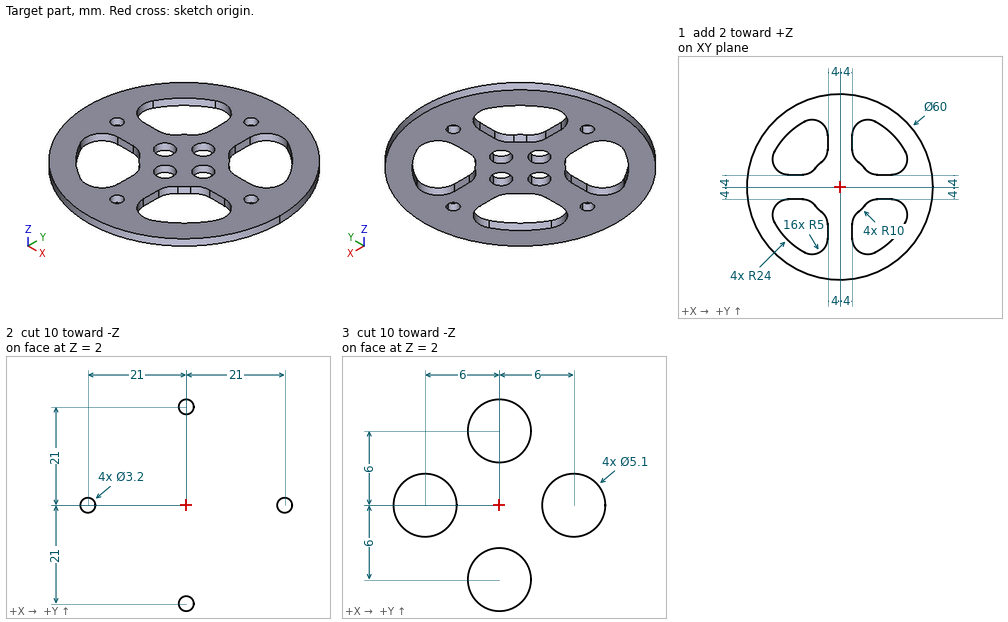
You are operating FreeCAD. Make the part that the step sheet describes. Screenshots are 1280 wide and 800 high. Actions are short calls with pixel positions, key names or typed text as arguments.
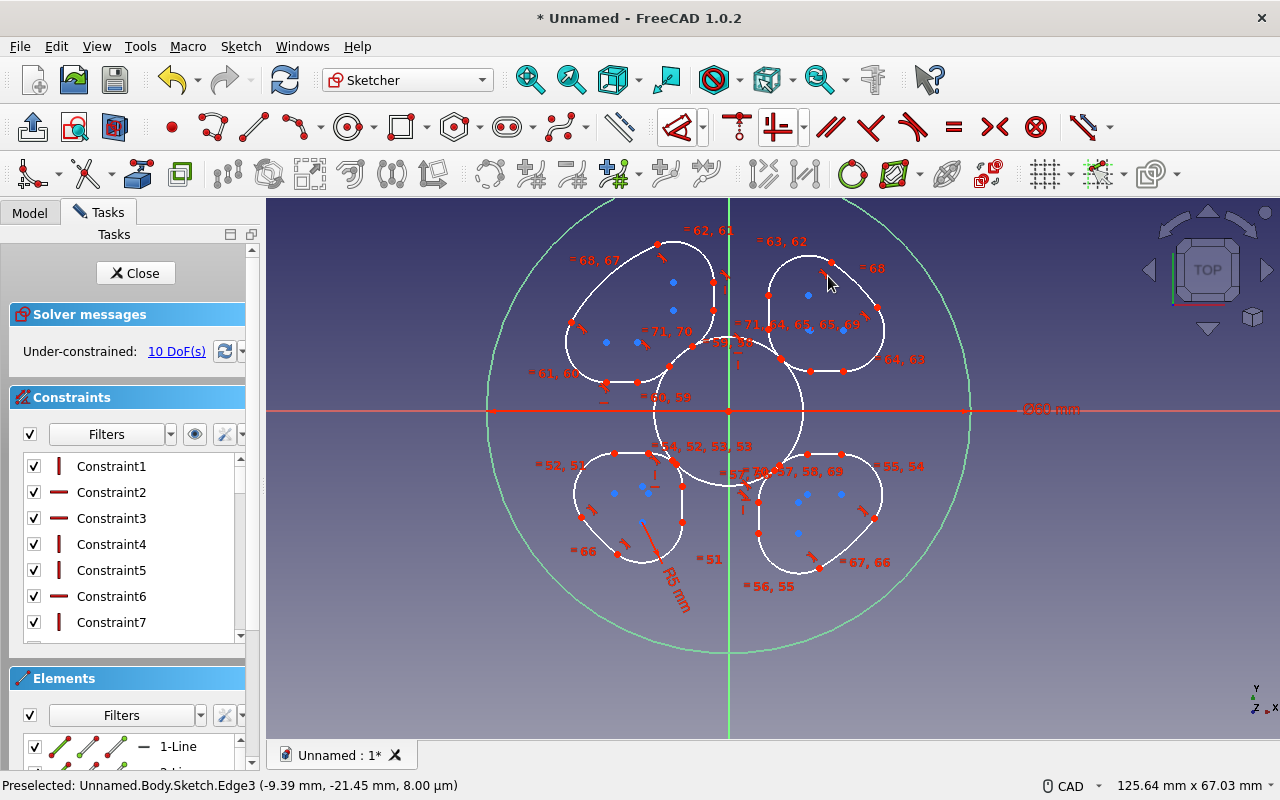
click(591, 529)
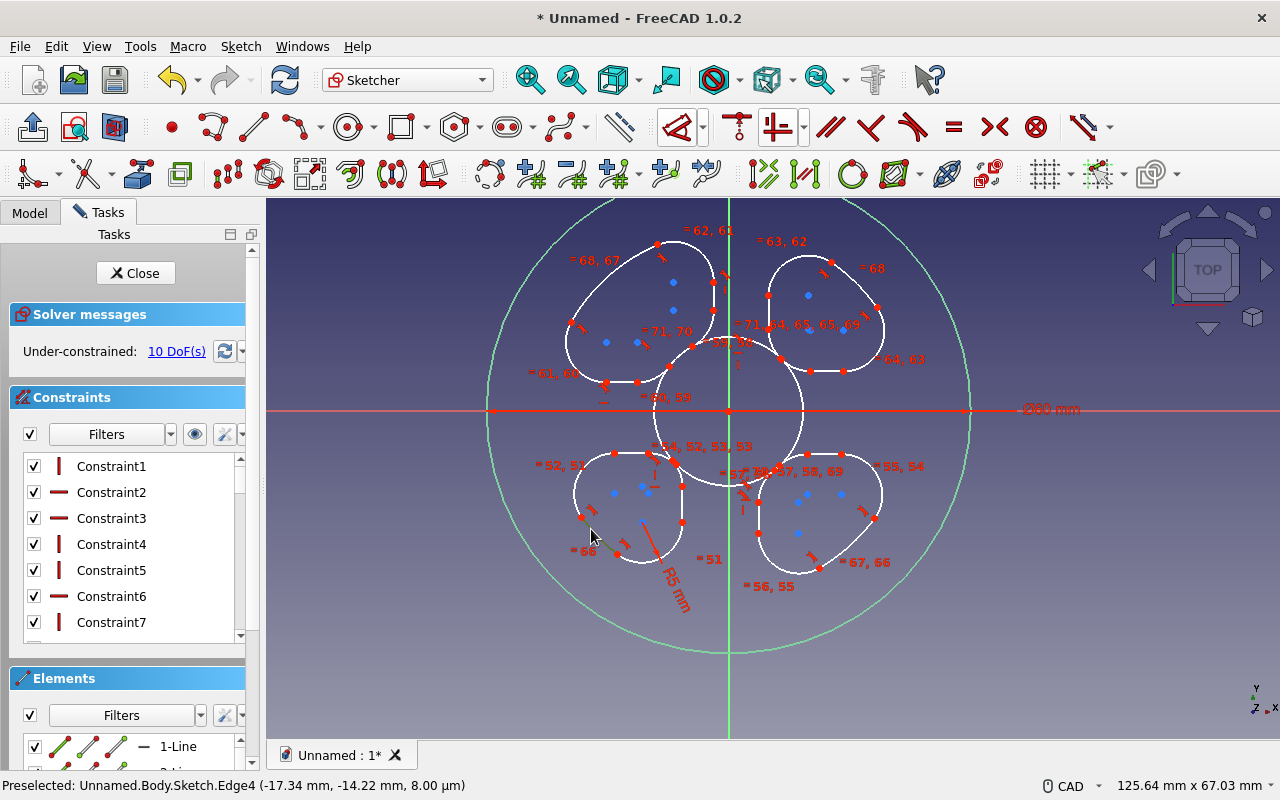
click(702, 128)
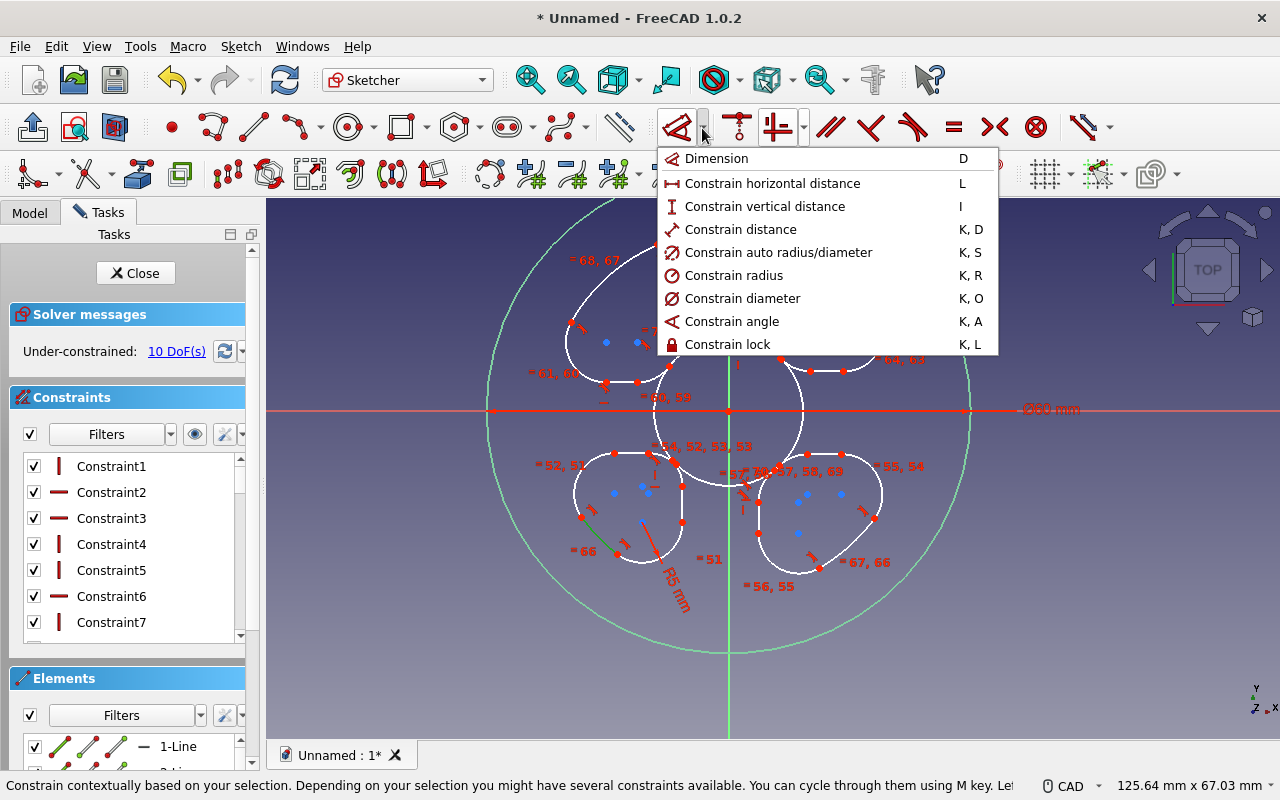
click(828, 276)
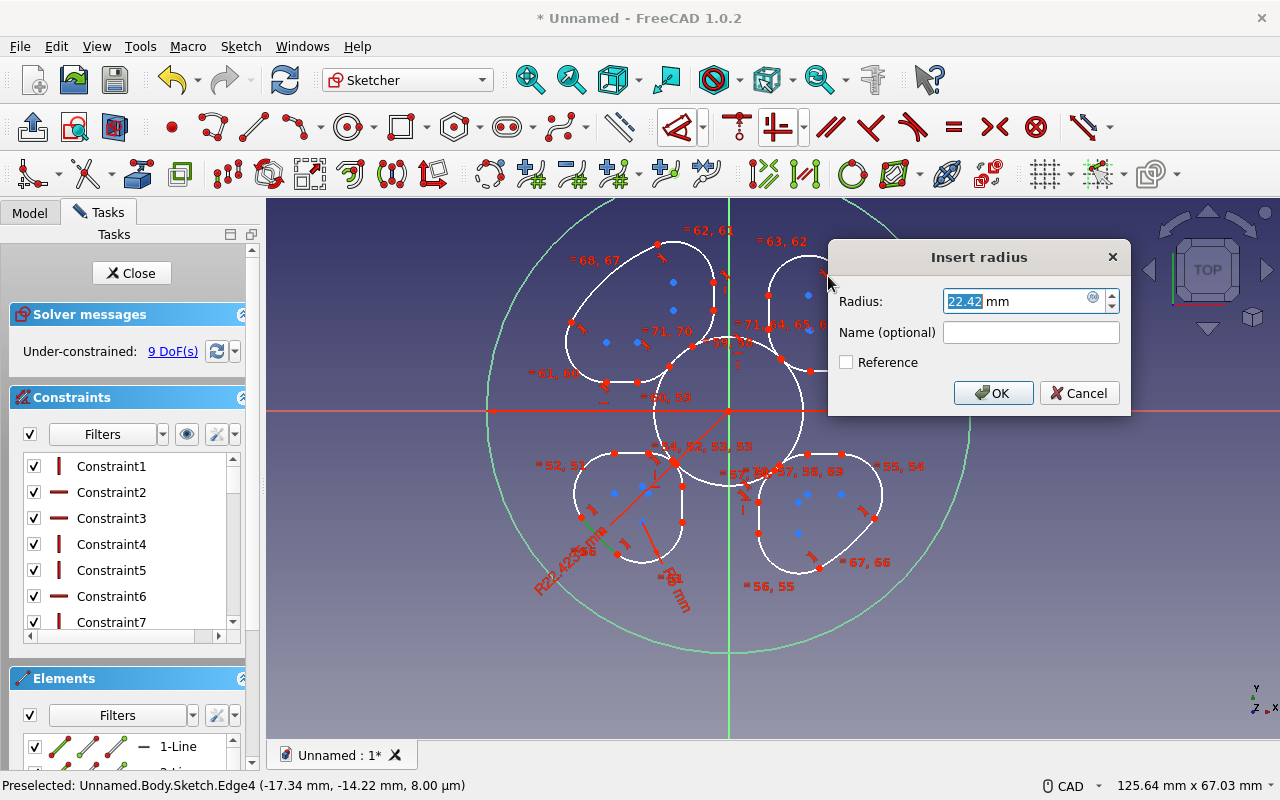
text(24)
key(Return)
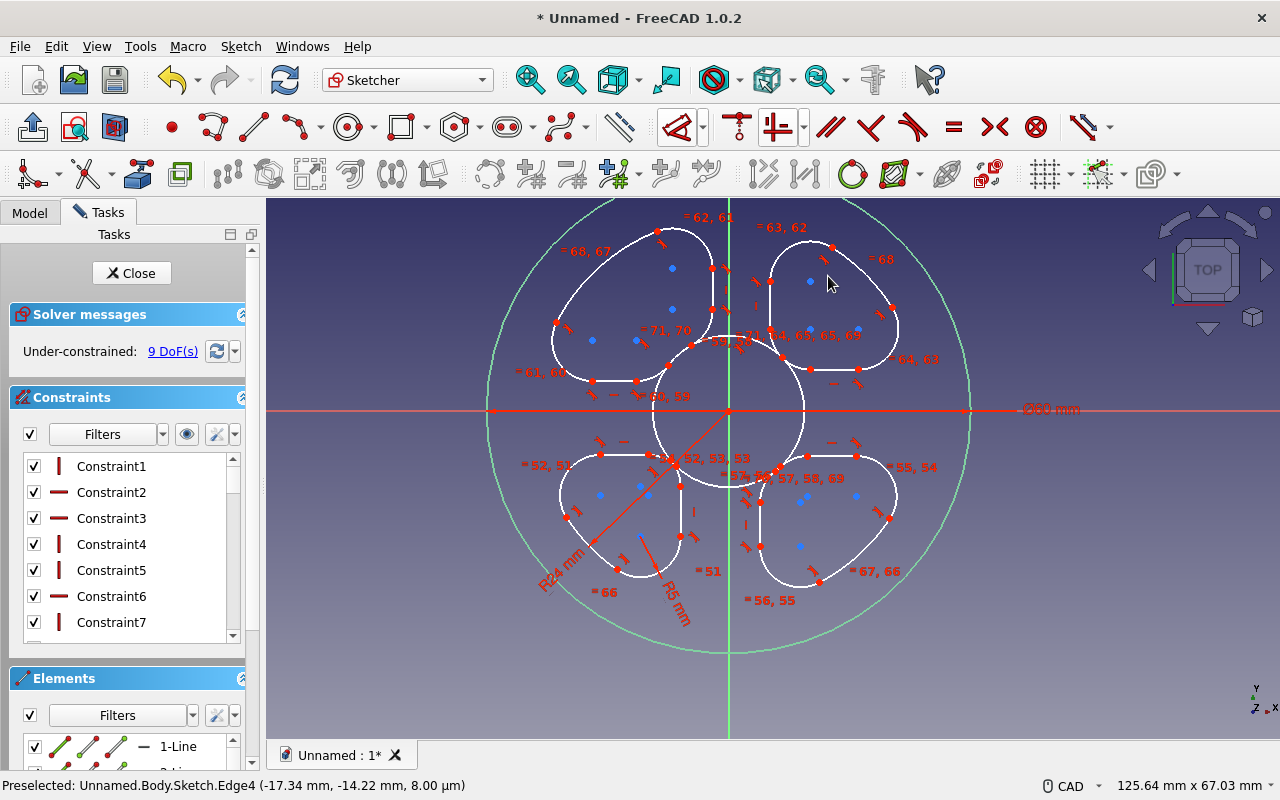
scroll(796, 446, up, 2)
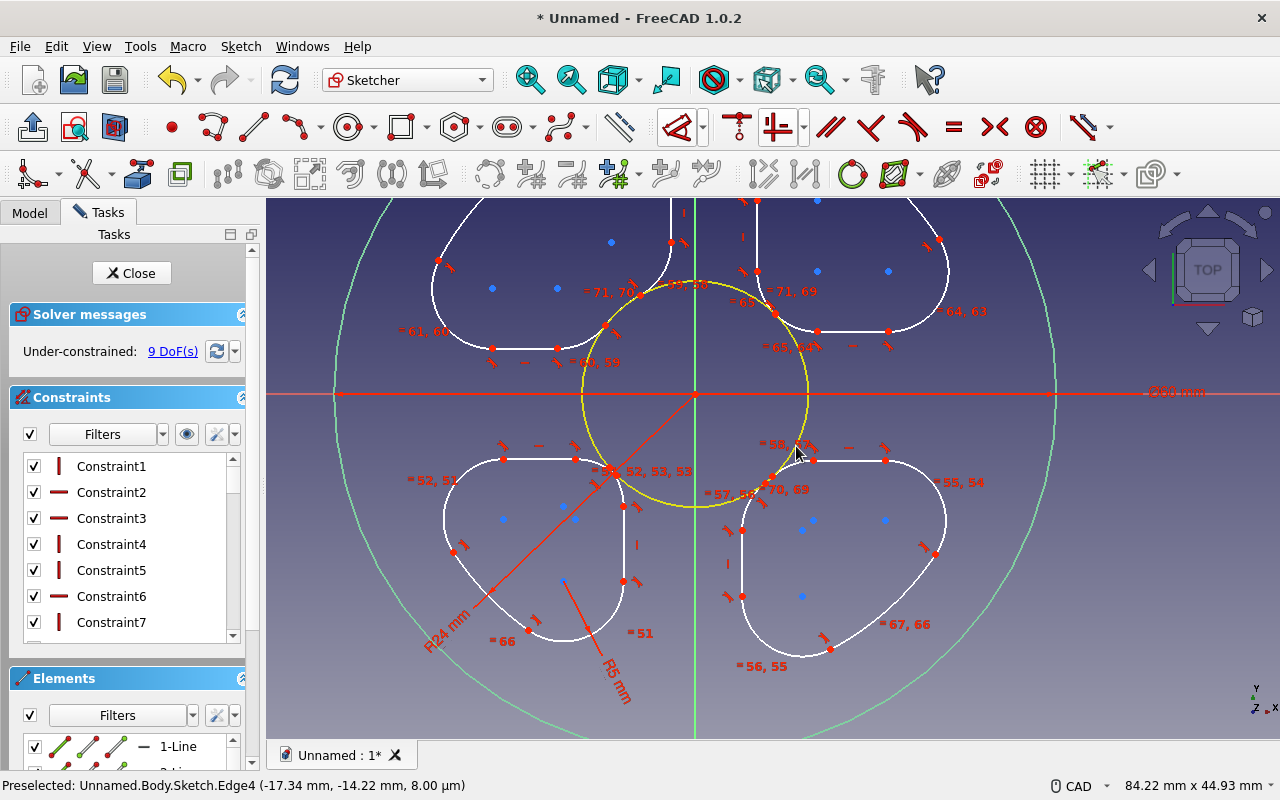
click(598, 337)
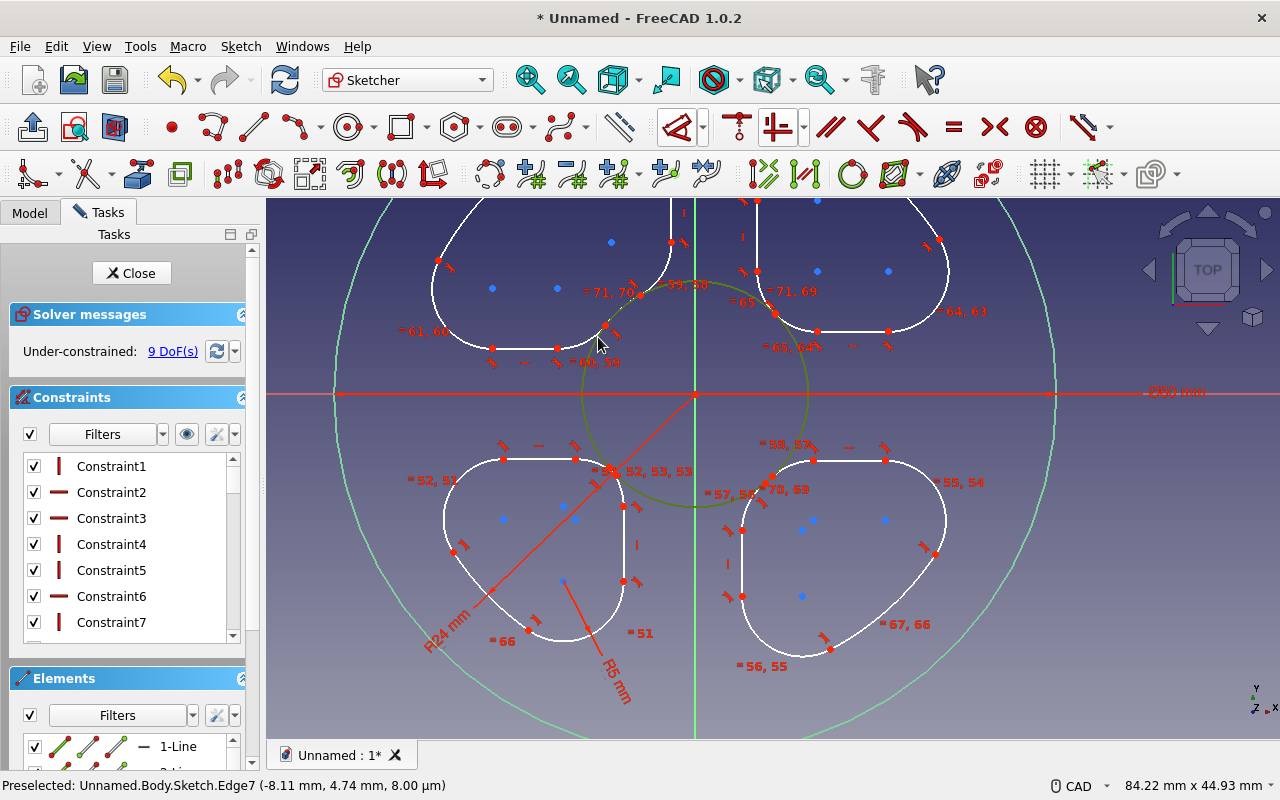
key(k)
key(r)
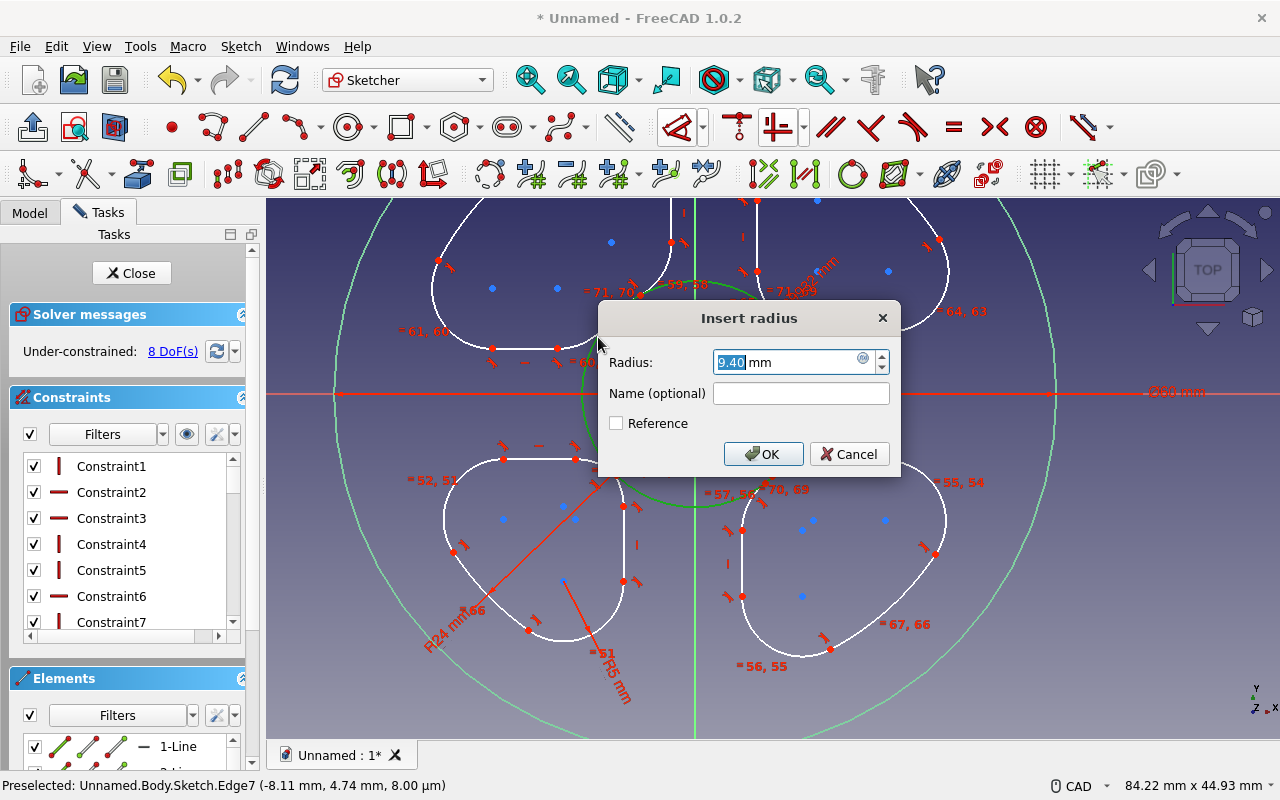
text(10)
key(Return)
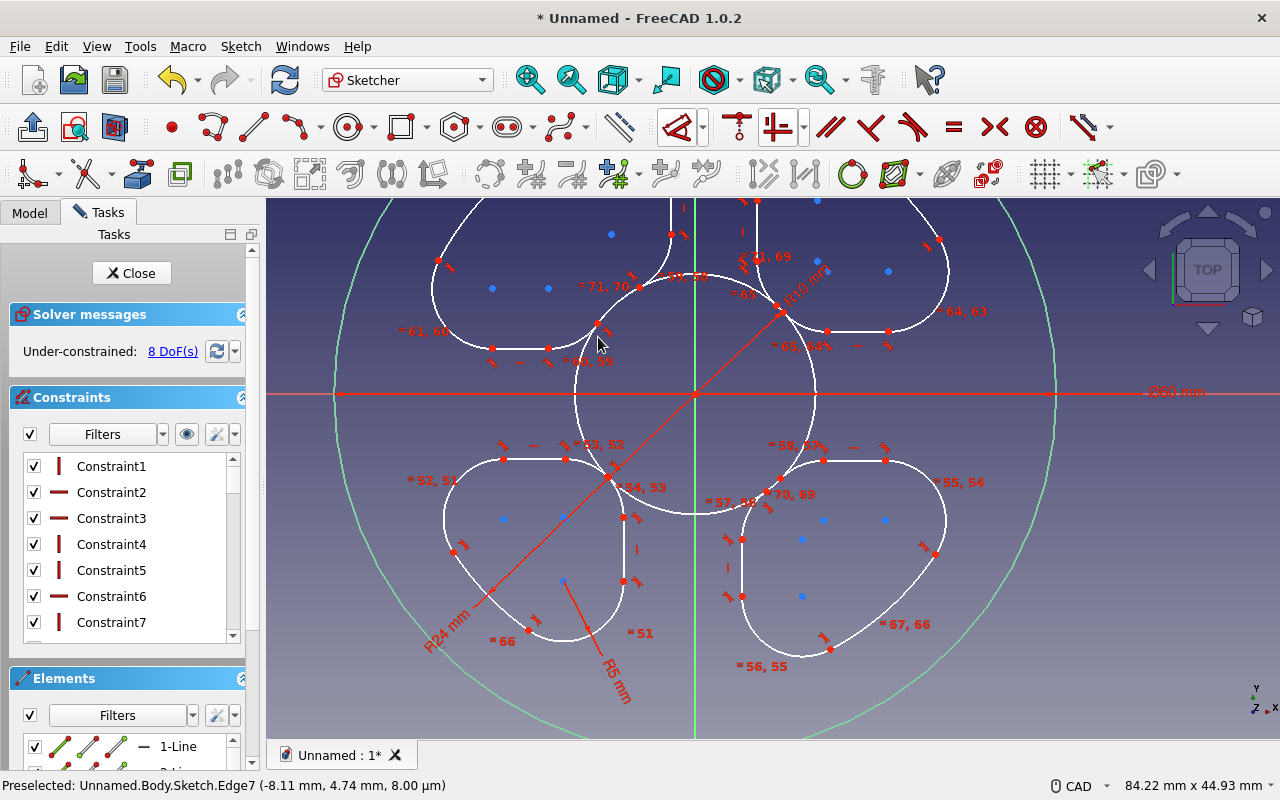
click(624, 518)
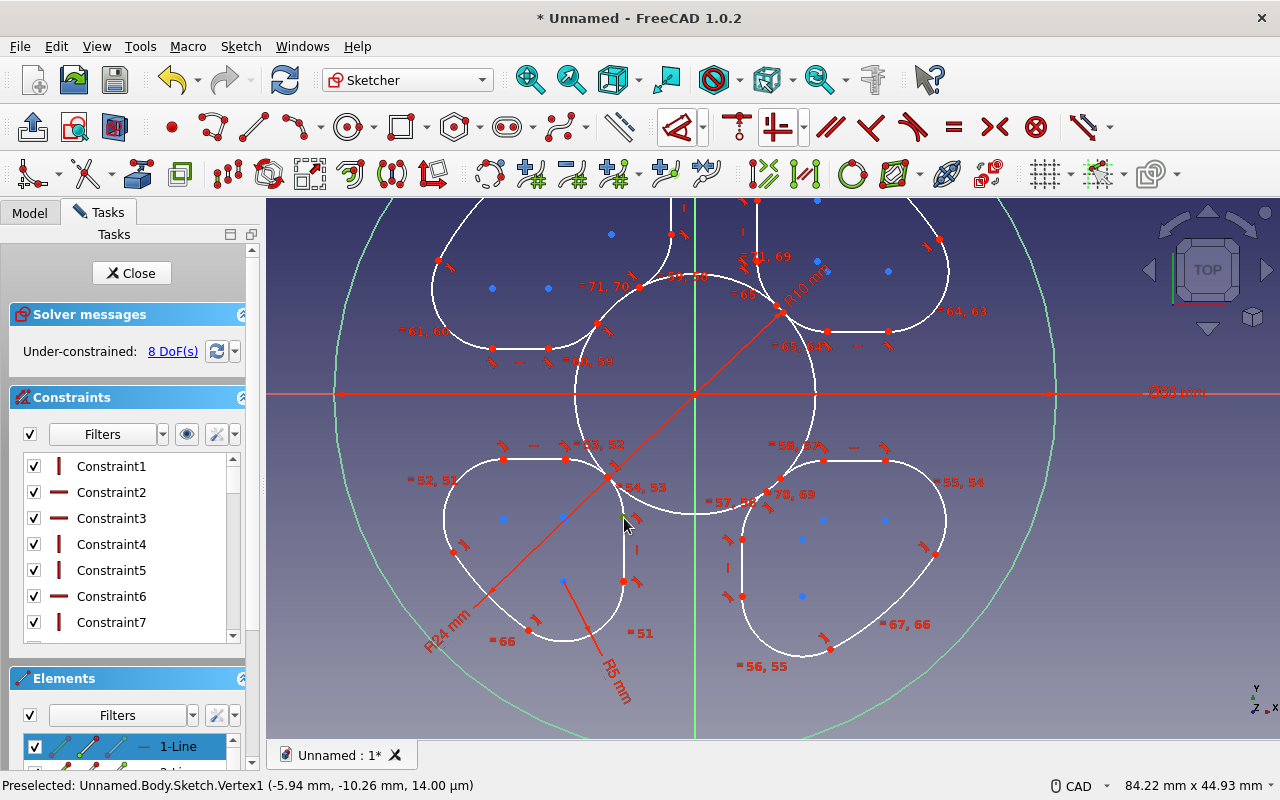
click(702, 128)